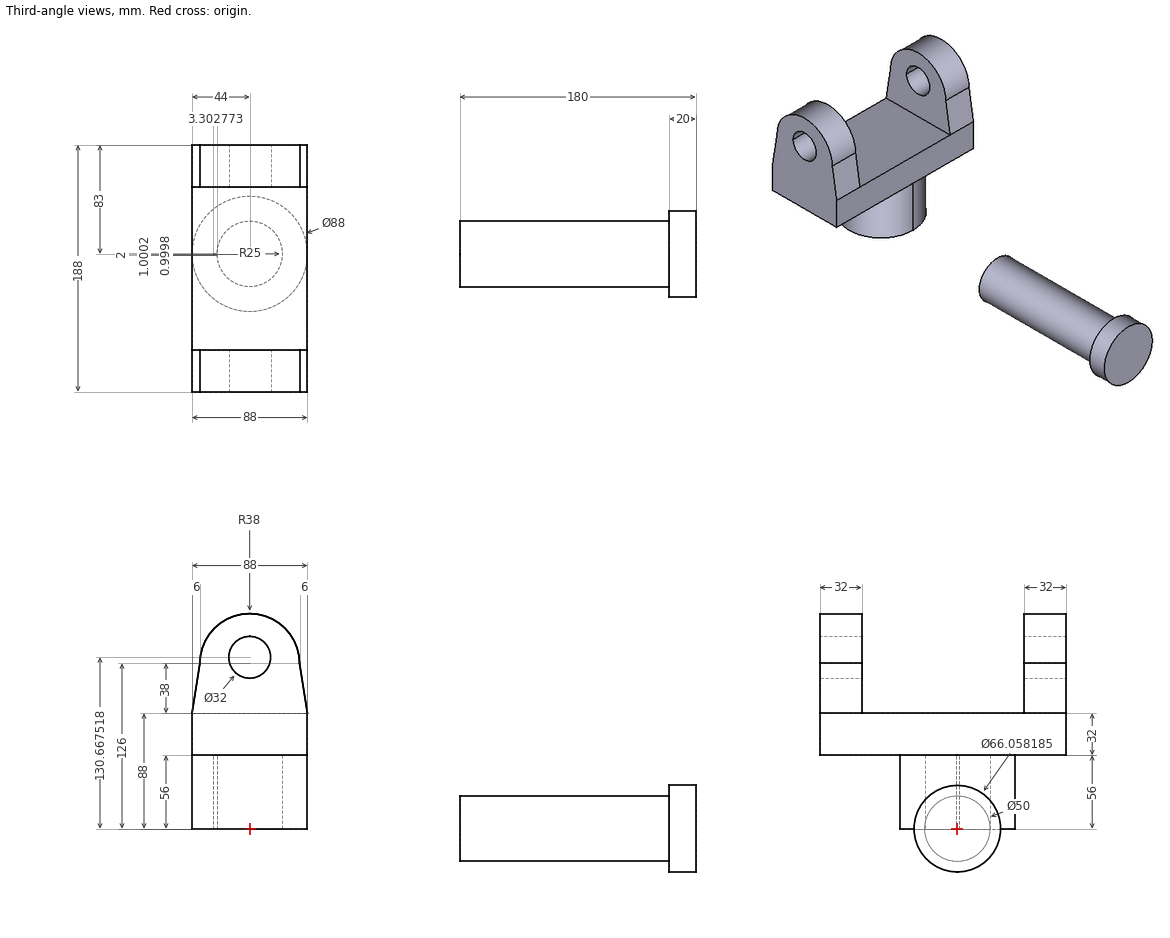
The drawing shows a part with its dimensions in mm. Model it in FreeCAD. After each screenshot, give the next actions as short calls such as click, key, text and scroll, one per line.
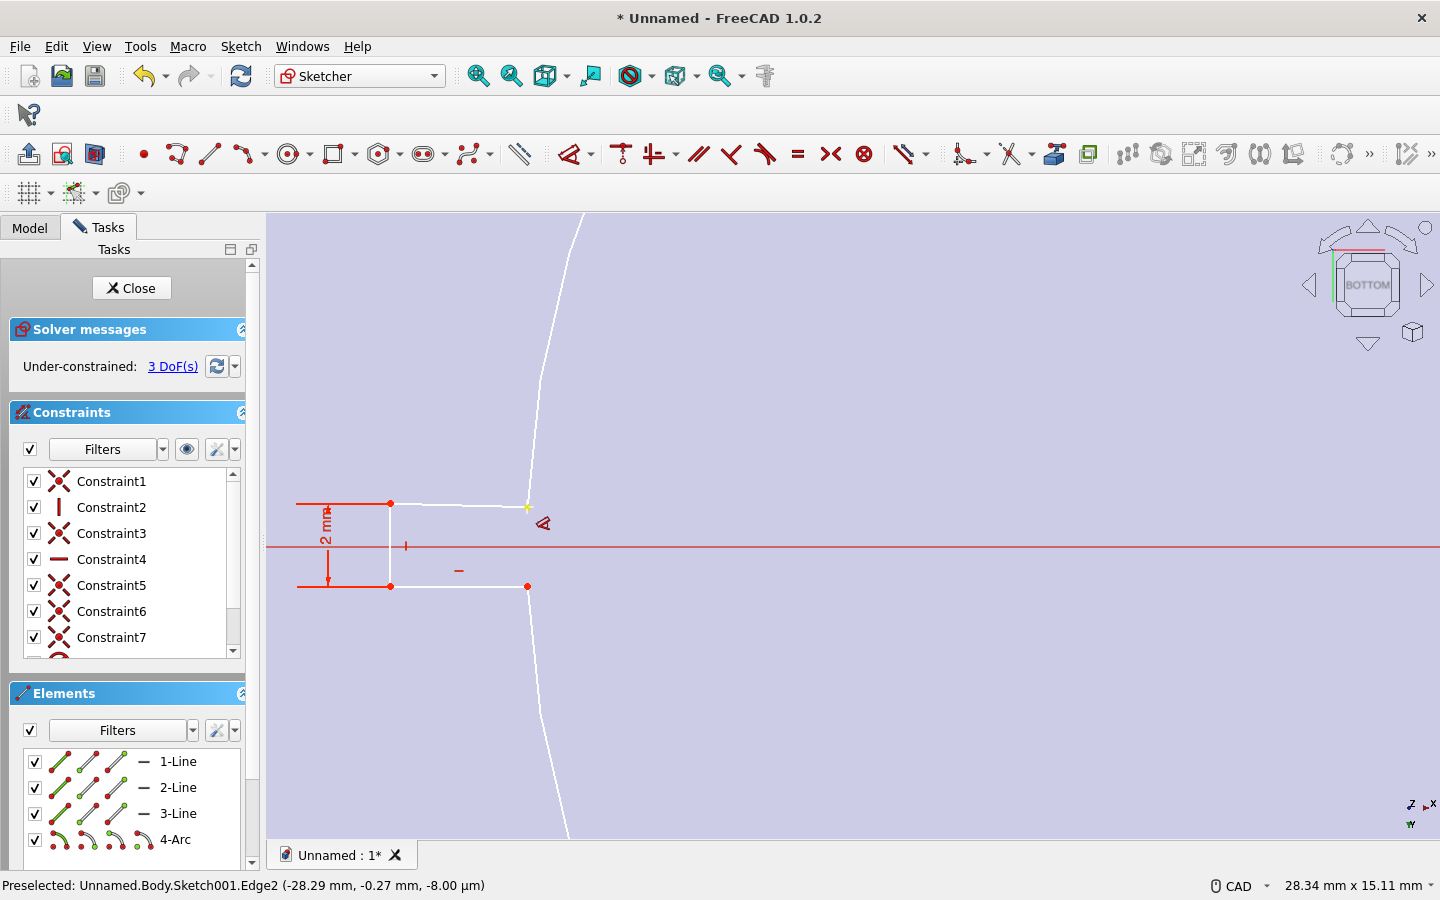
click(528, 507)
click(494, 527)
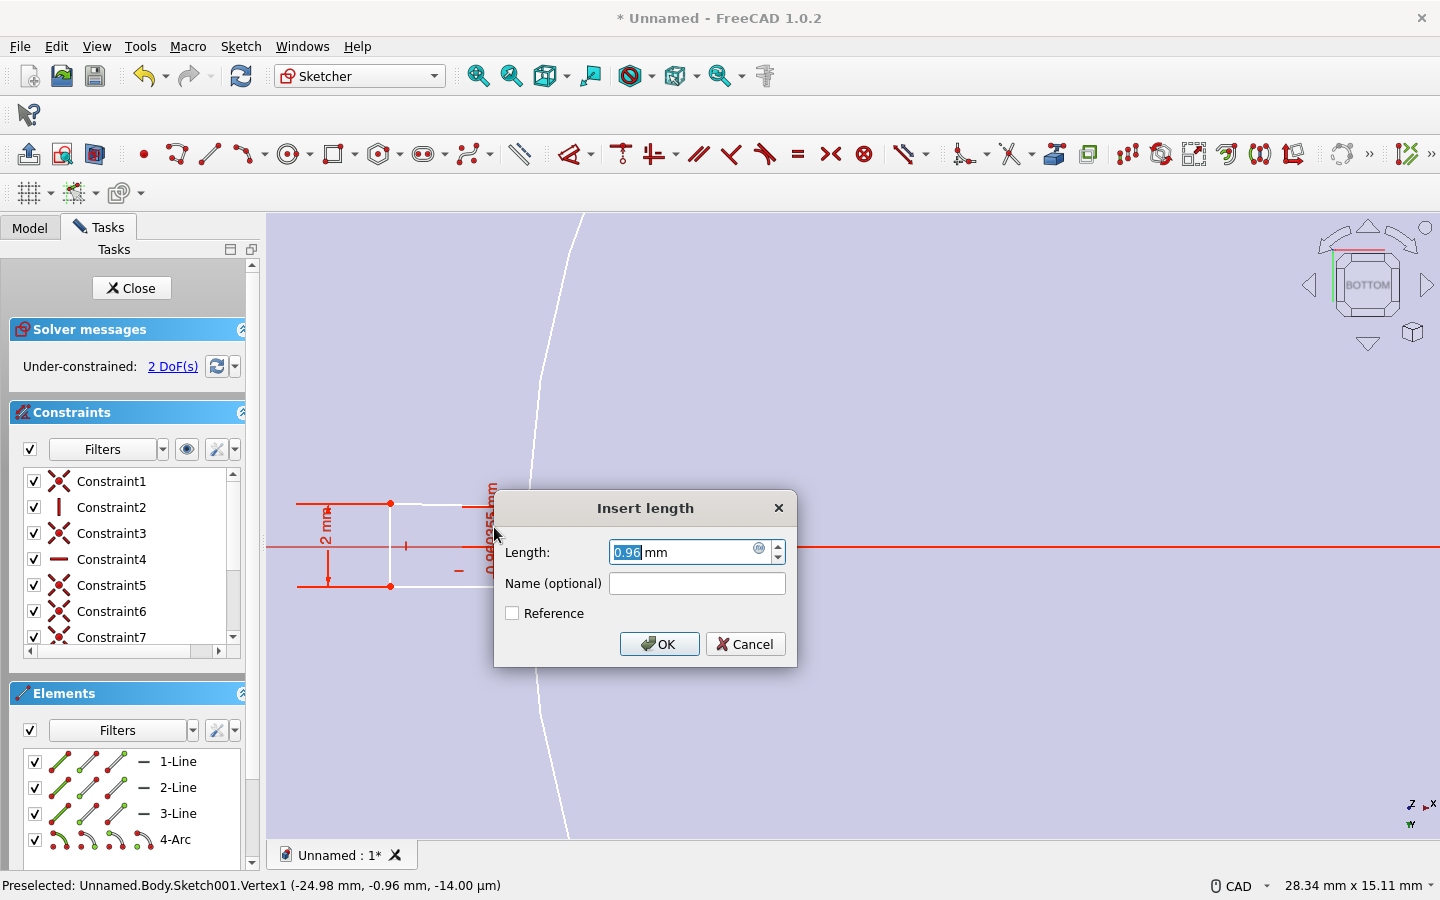
text(0.9998)
key(Return)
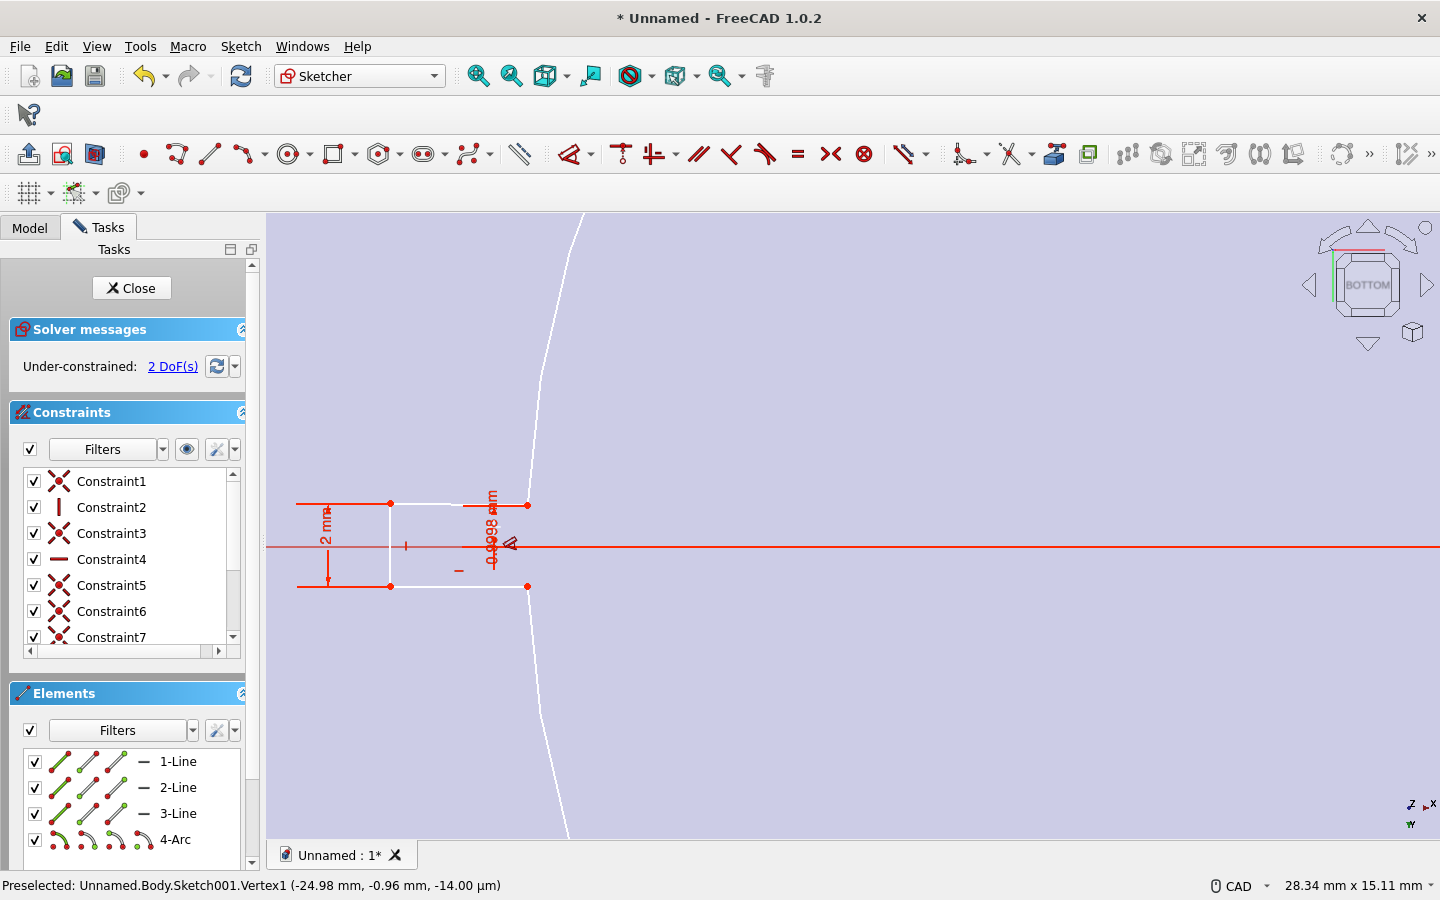
click(390, 504)
click(356, 535)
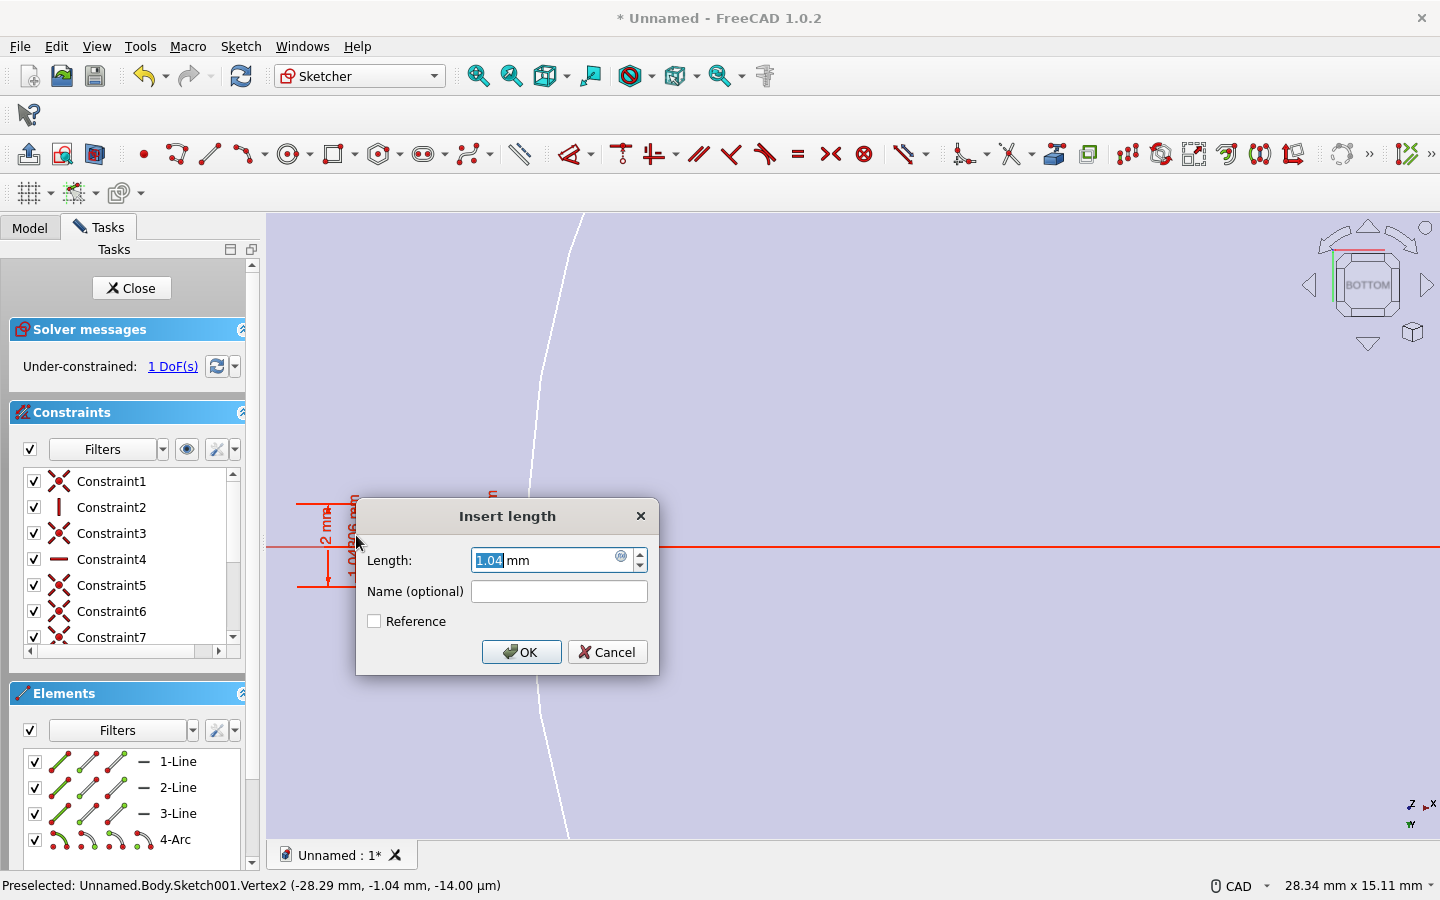
text(1.0002)
key(Return)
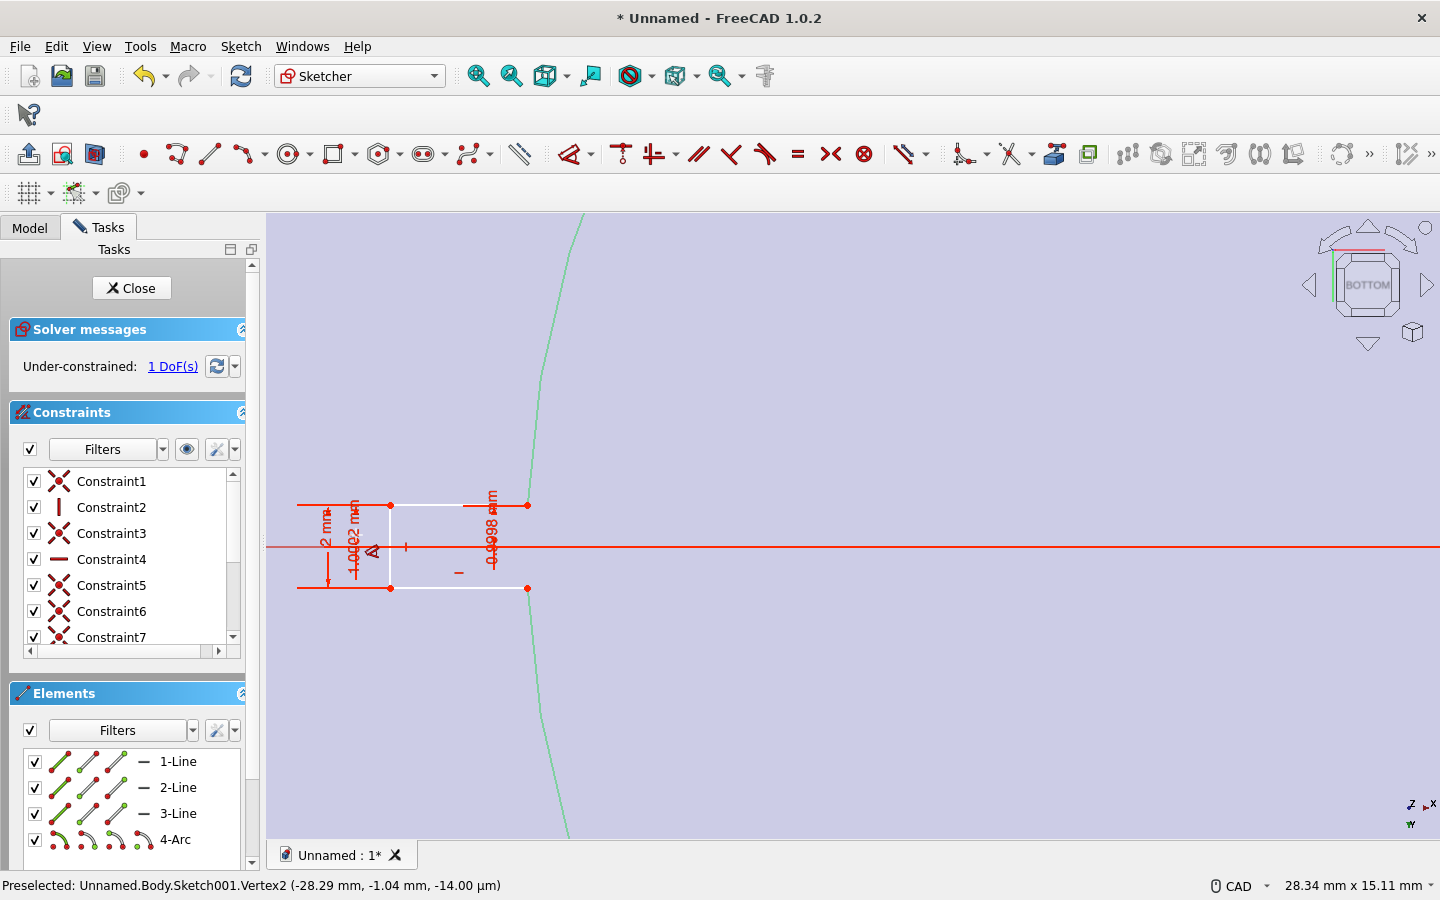
click(432, 588)
click(459, 622)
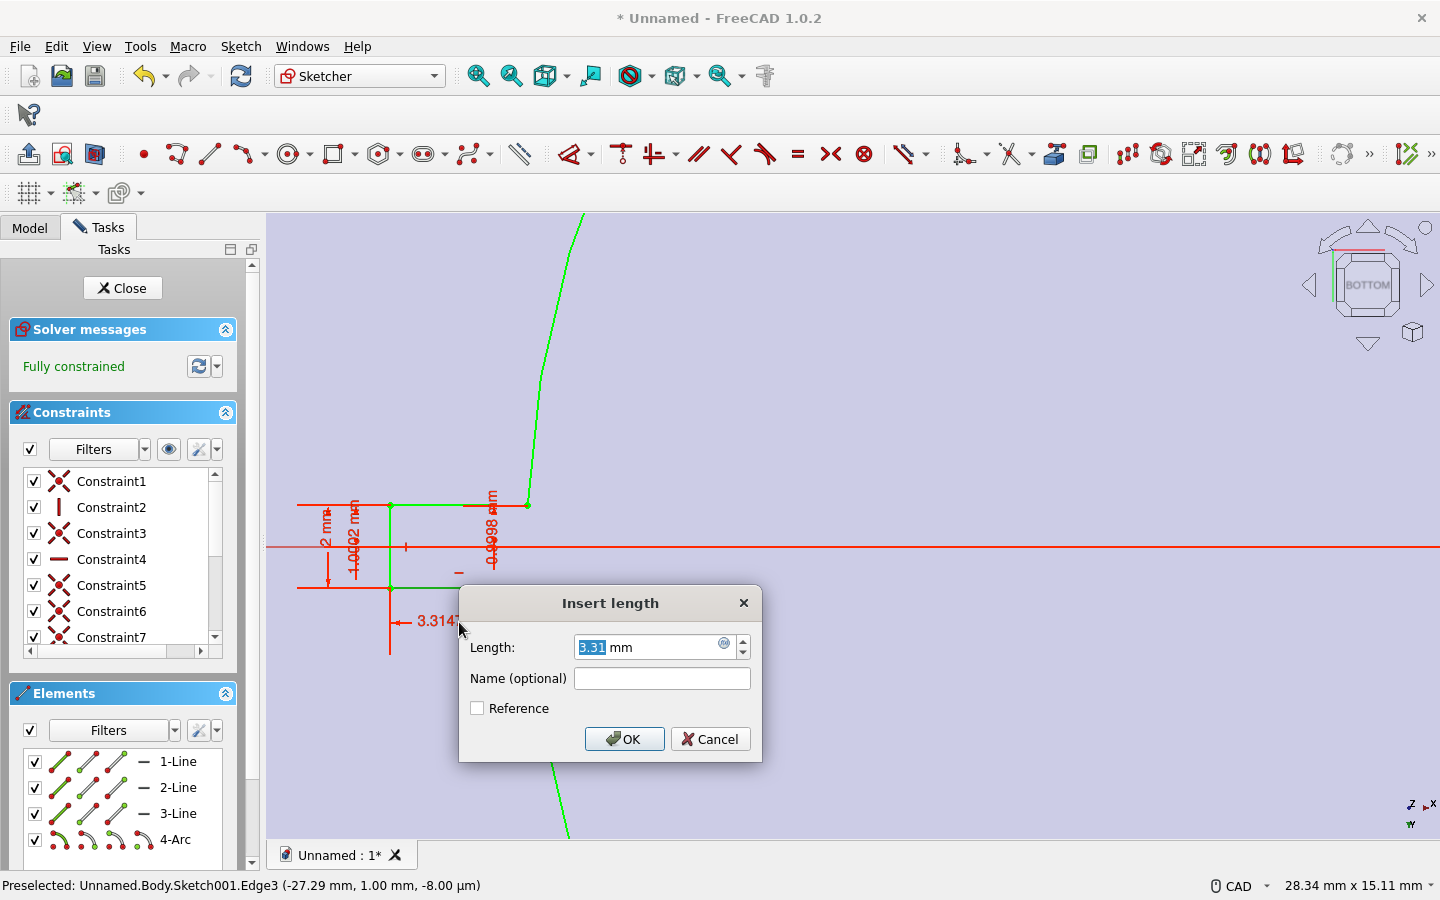
text(3.302773)
key(Return)
key(Escape)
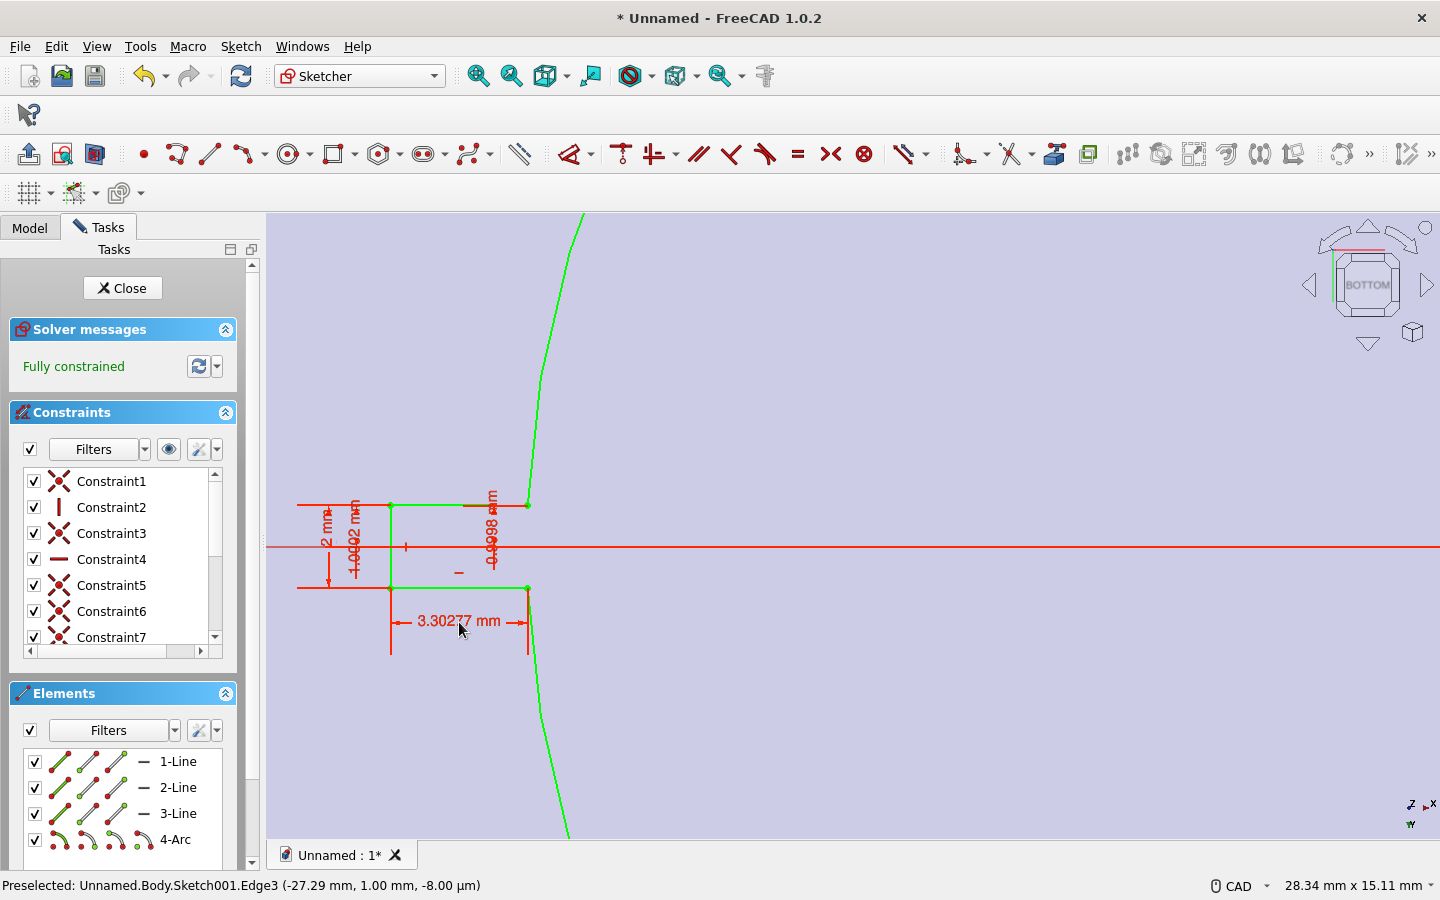
click(123, 288)